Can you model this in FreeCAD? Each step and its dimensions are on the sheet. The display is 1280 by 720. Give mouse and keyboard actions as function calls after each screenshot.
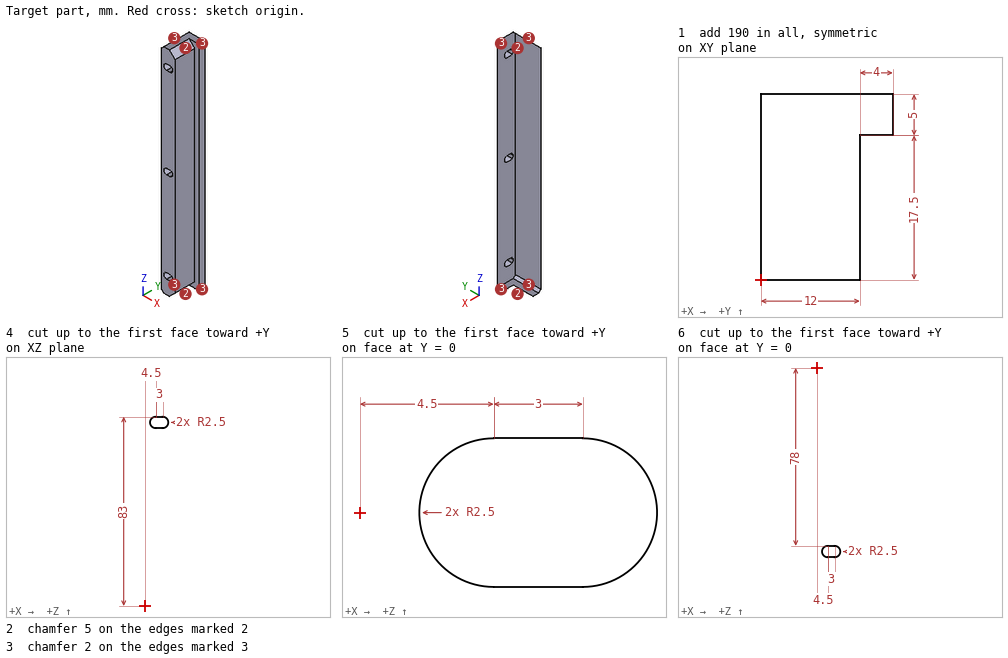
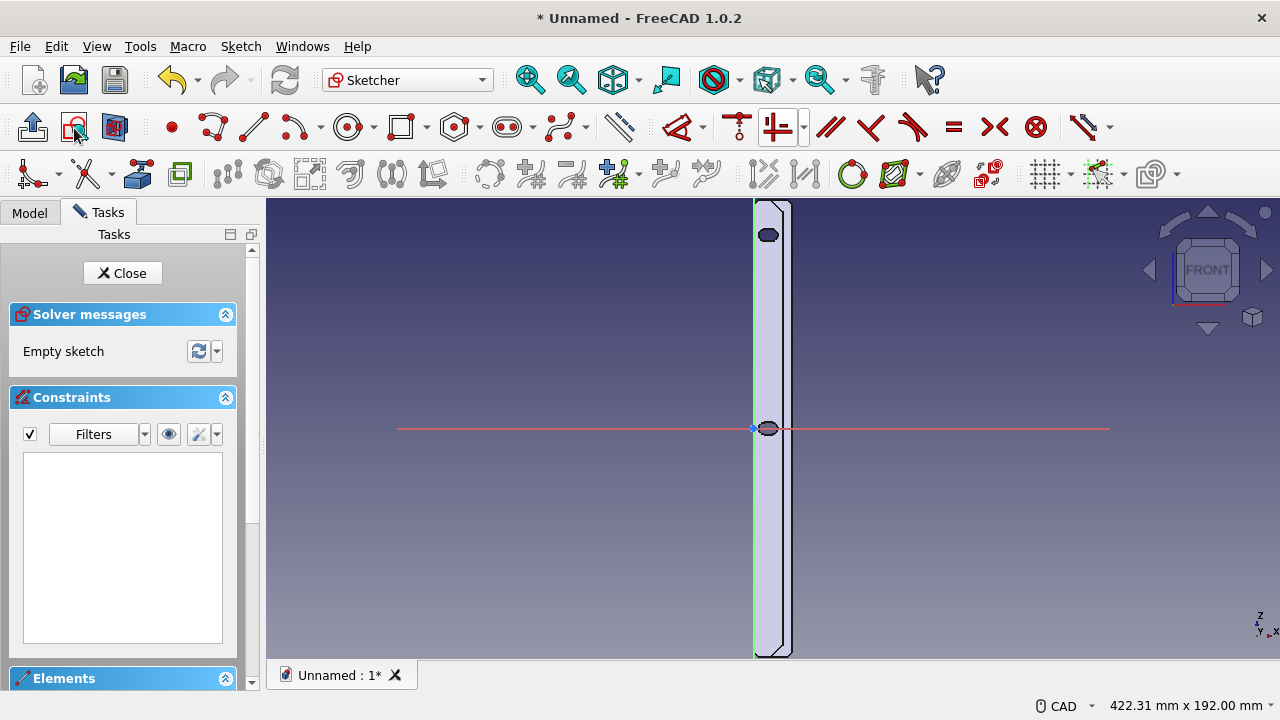
scroll(772, 631, up, 15)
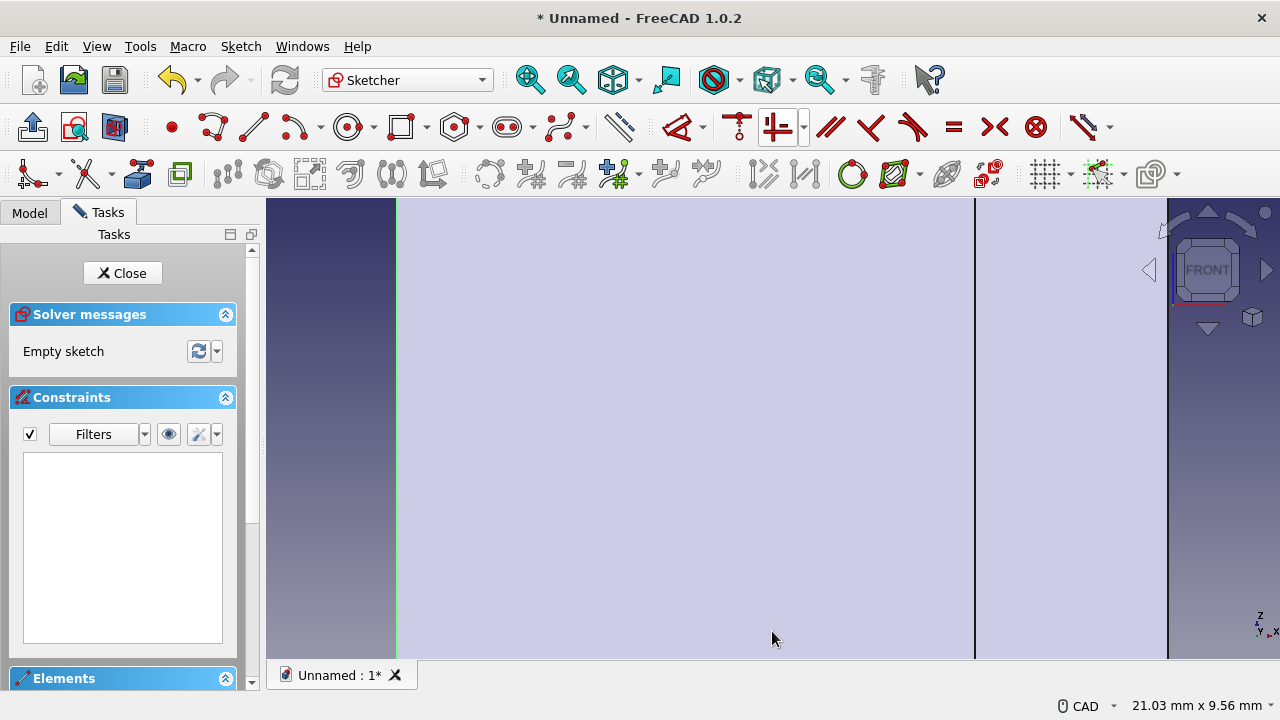
click(506, 128)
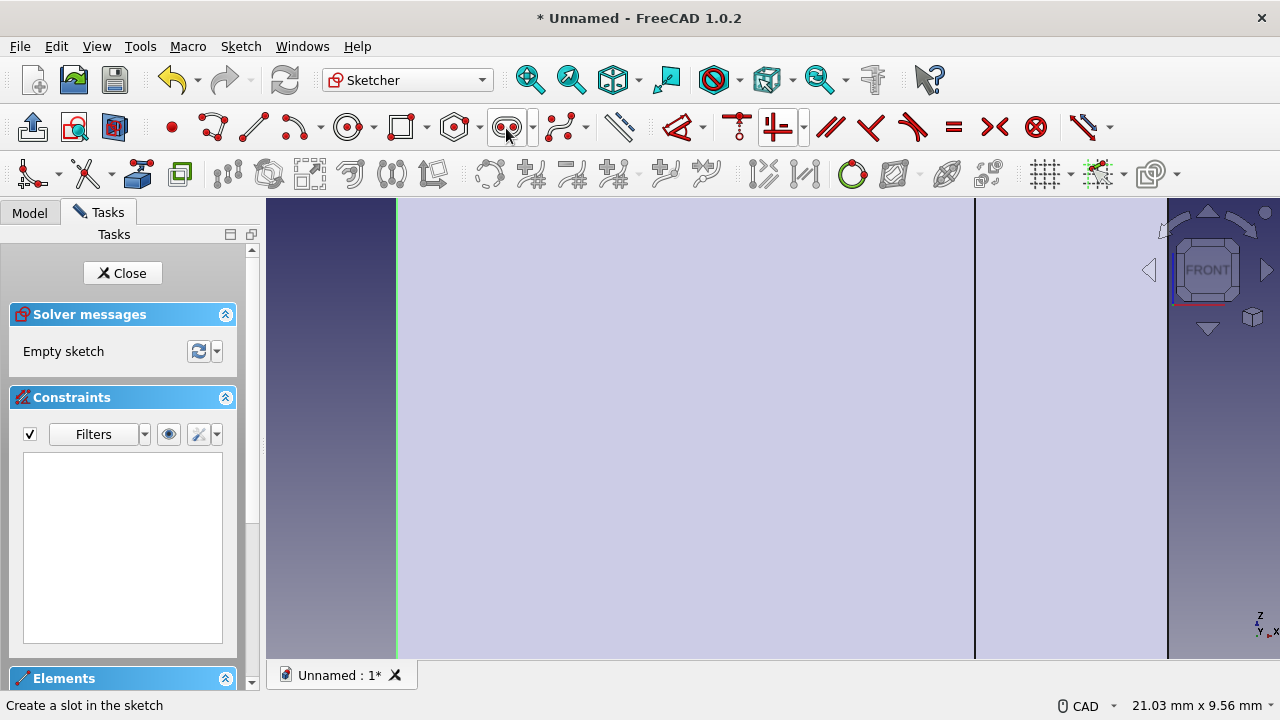
click(614, 428)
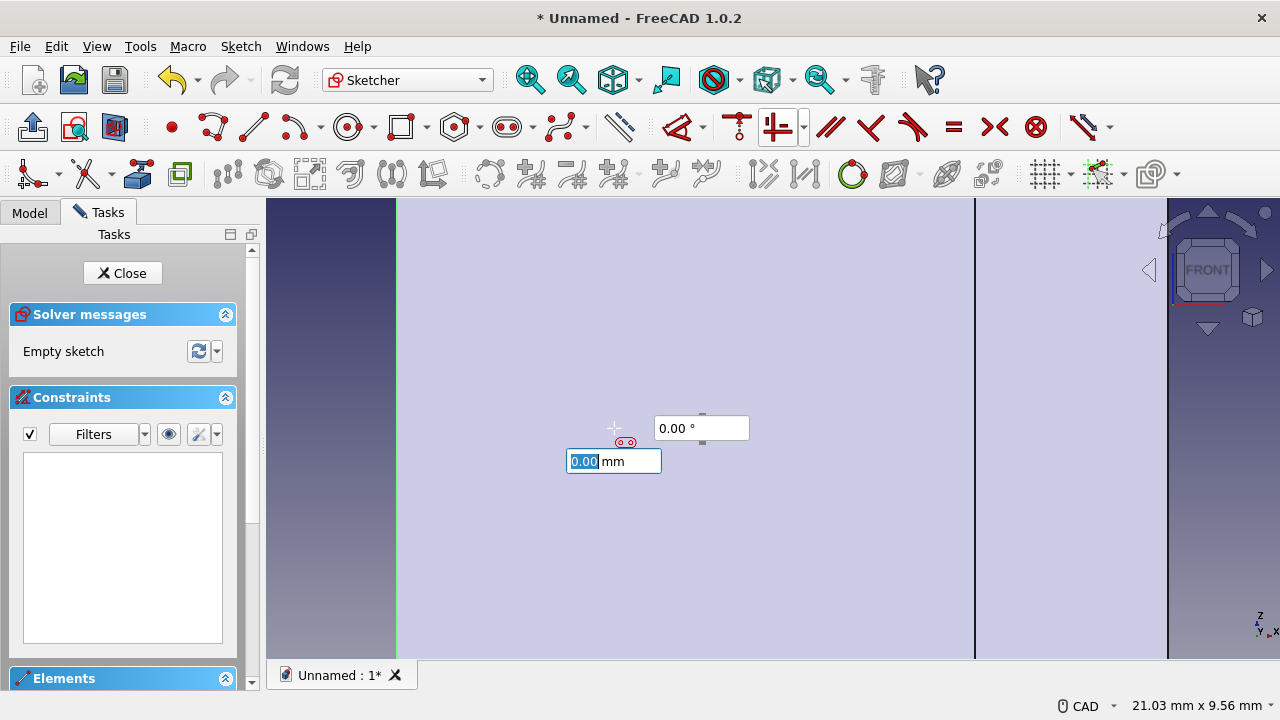
click(758, 428)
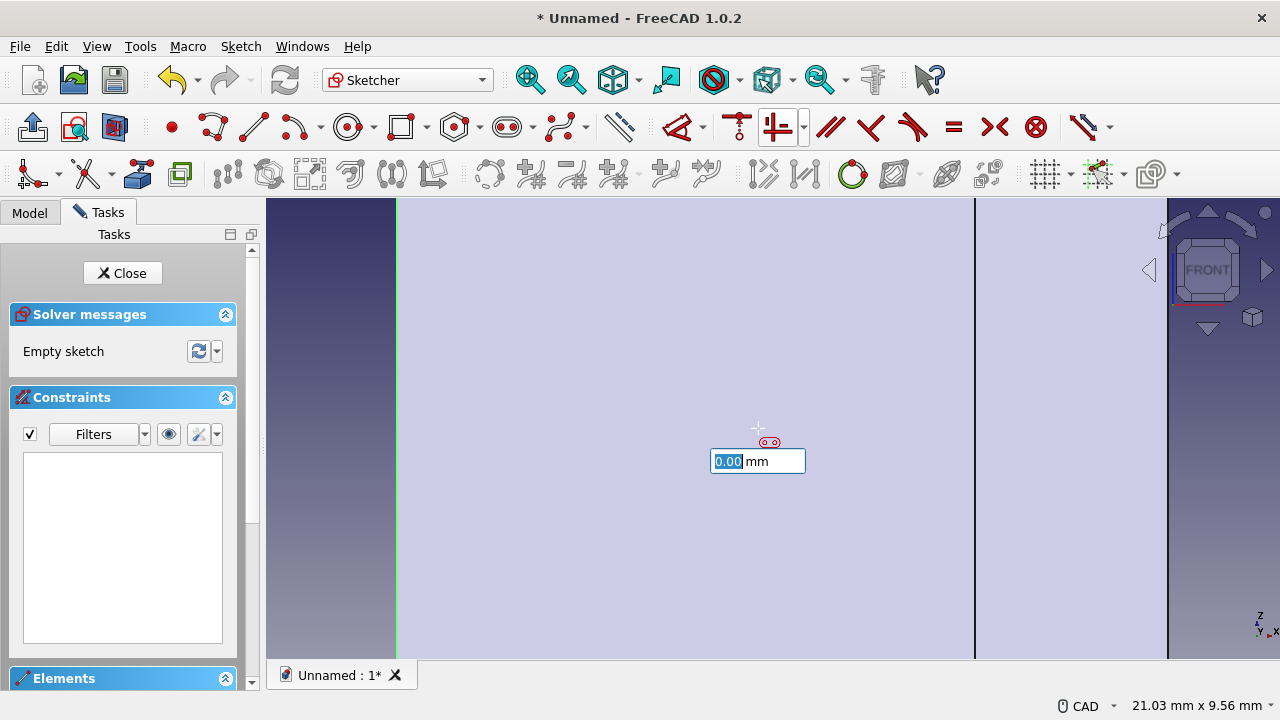
click(686, 549)
key(Escape)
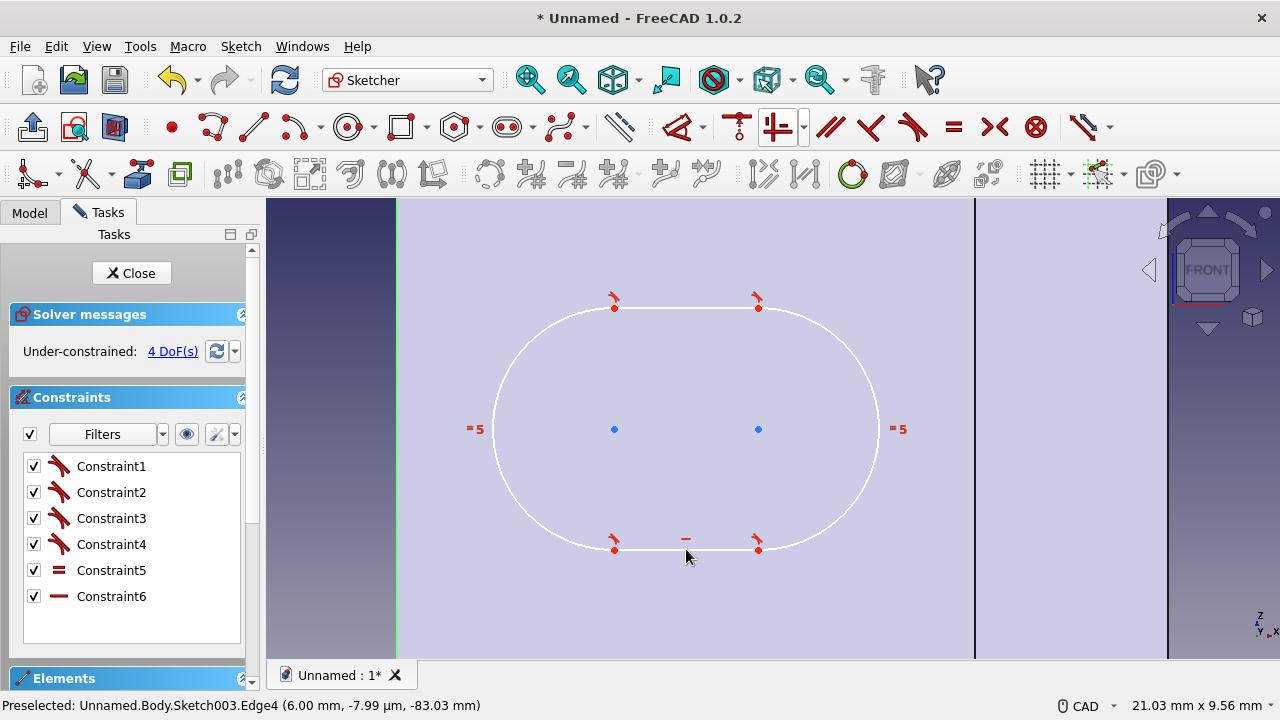
click(676, 128)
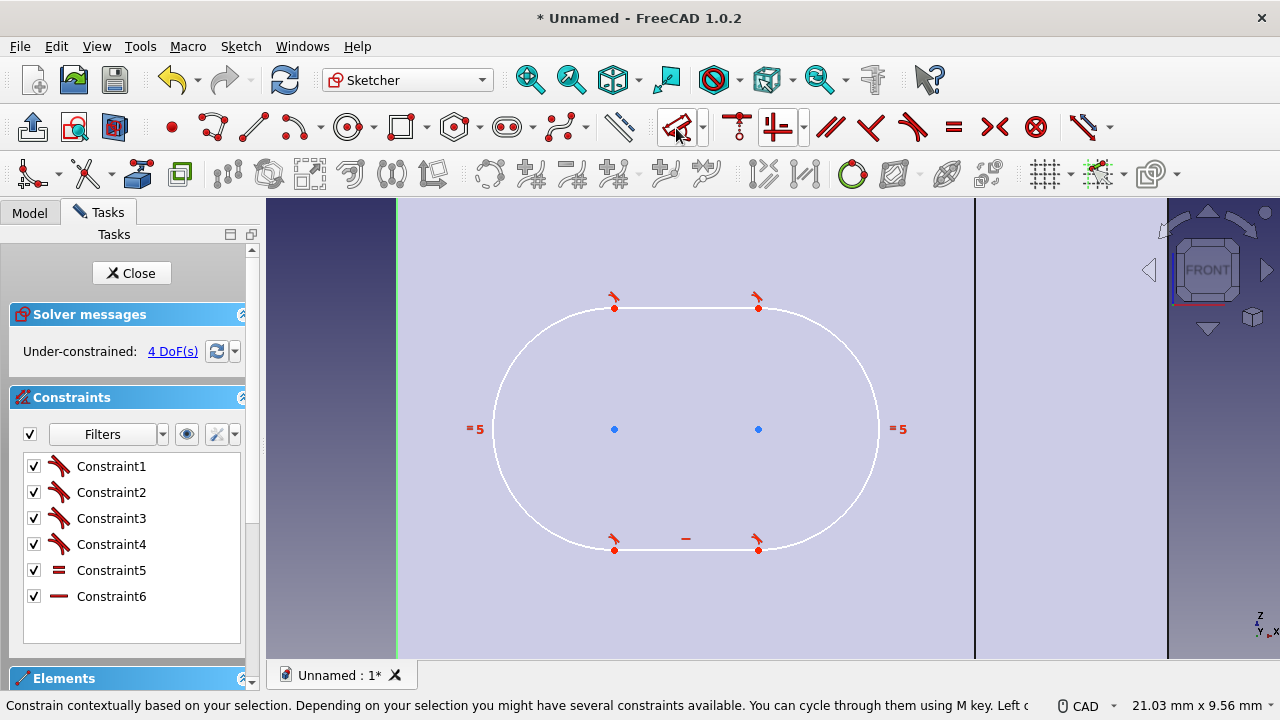
click(516, 358)
click(490, 339)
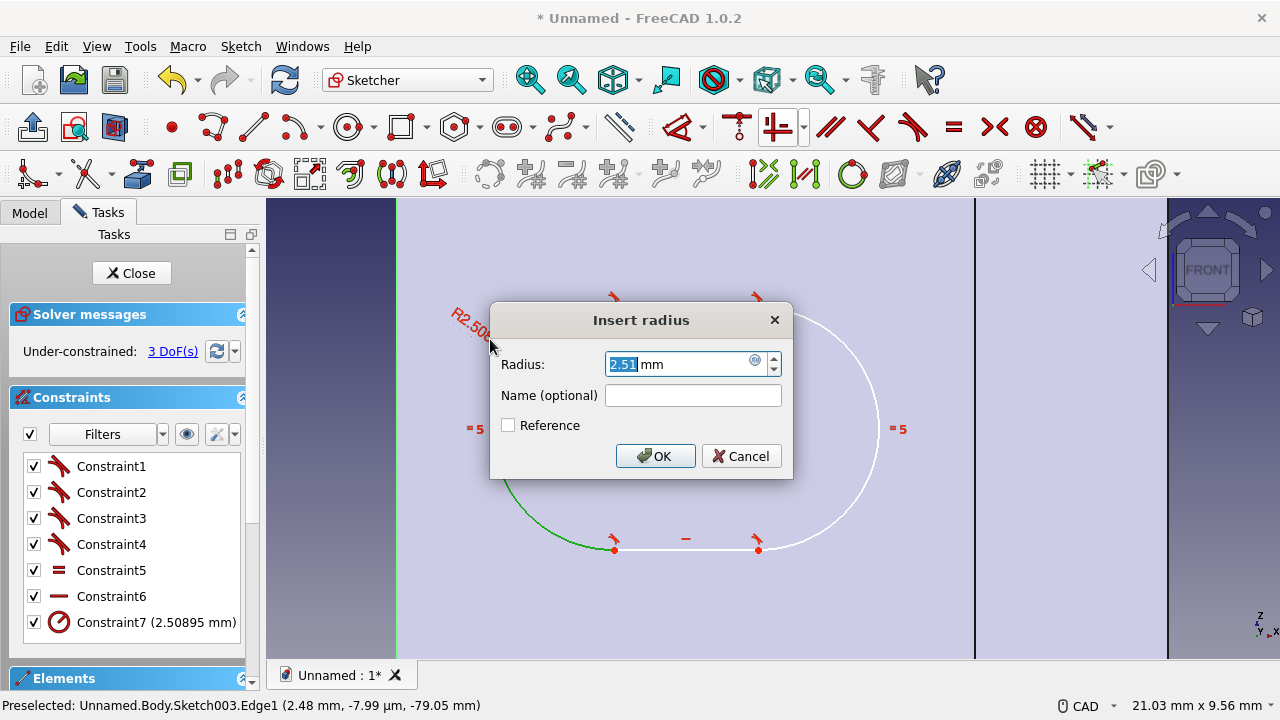
text(2.5)
key(Return)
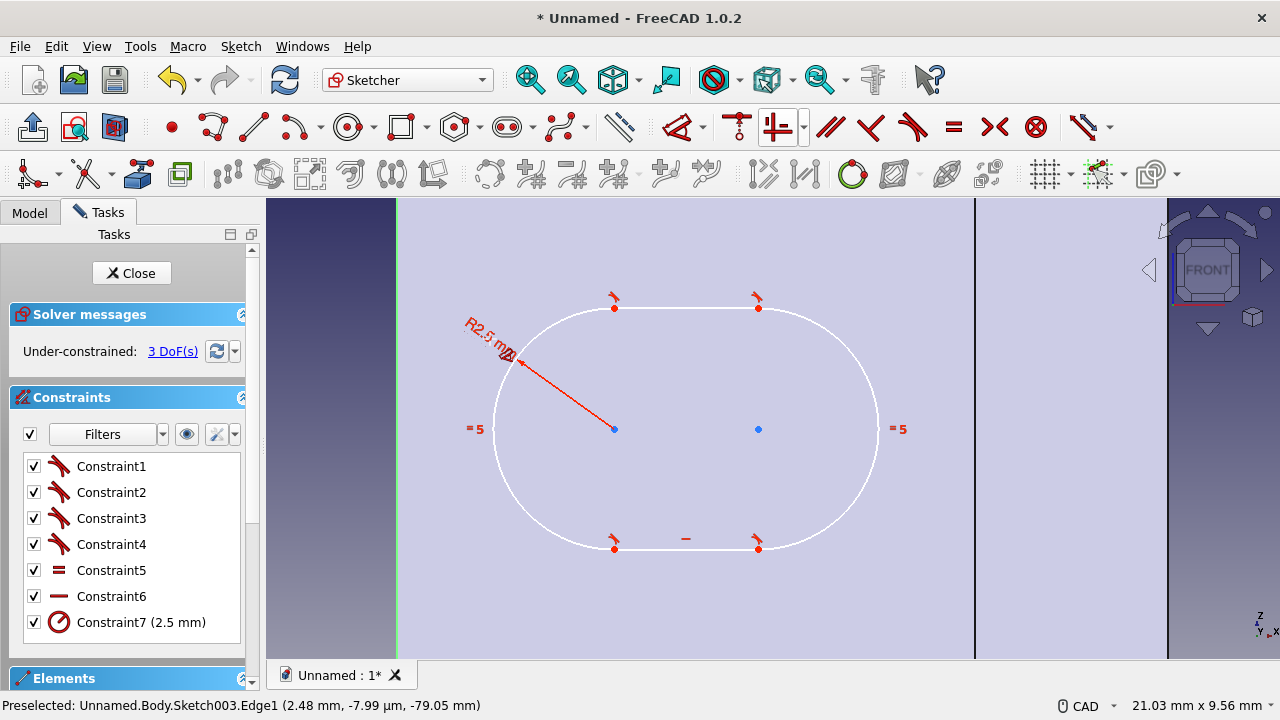
click(657, 308)
click(686, 274)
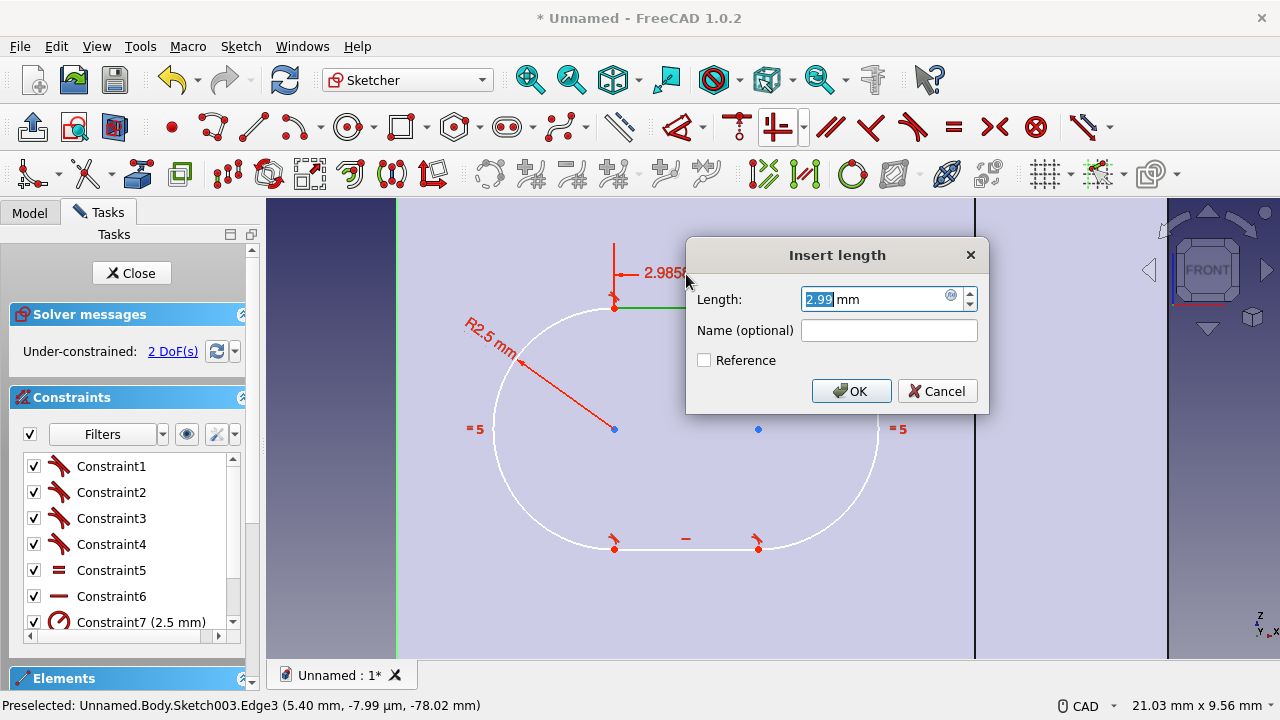
text(3)
key(Return)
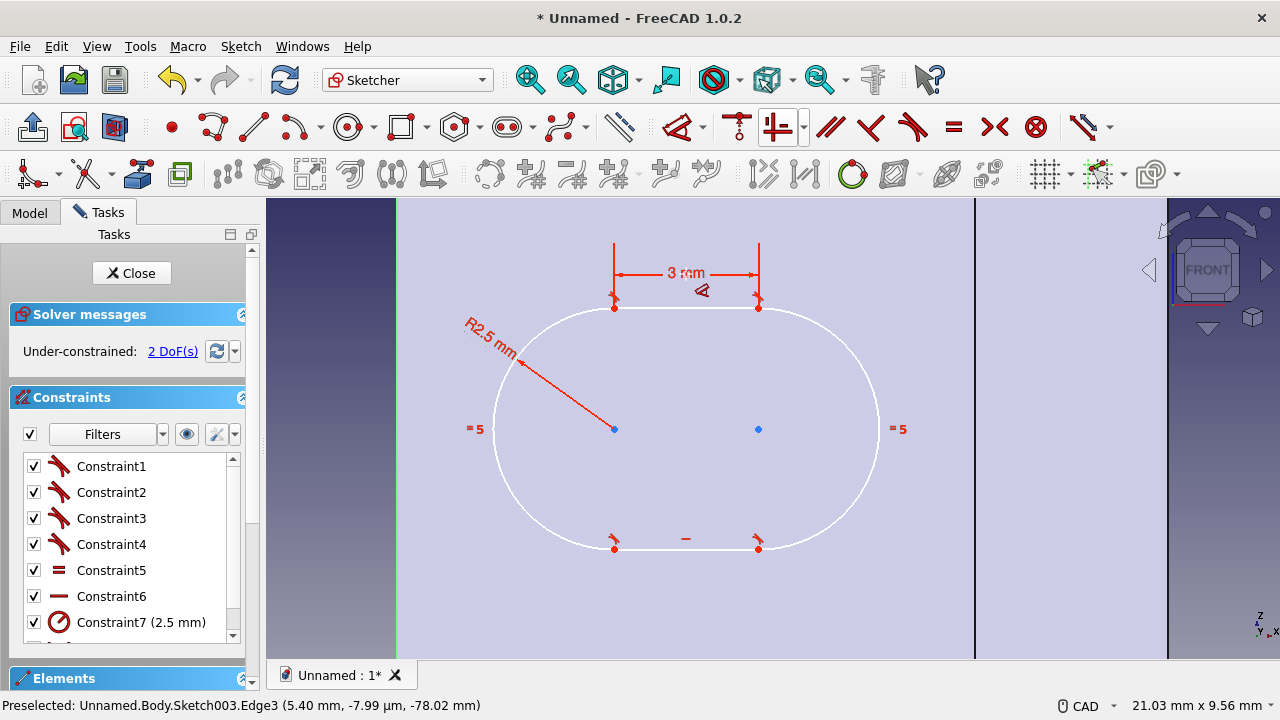
click(614, 308)
click(363, 267)